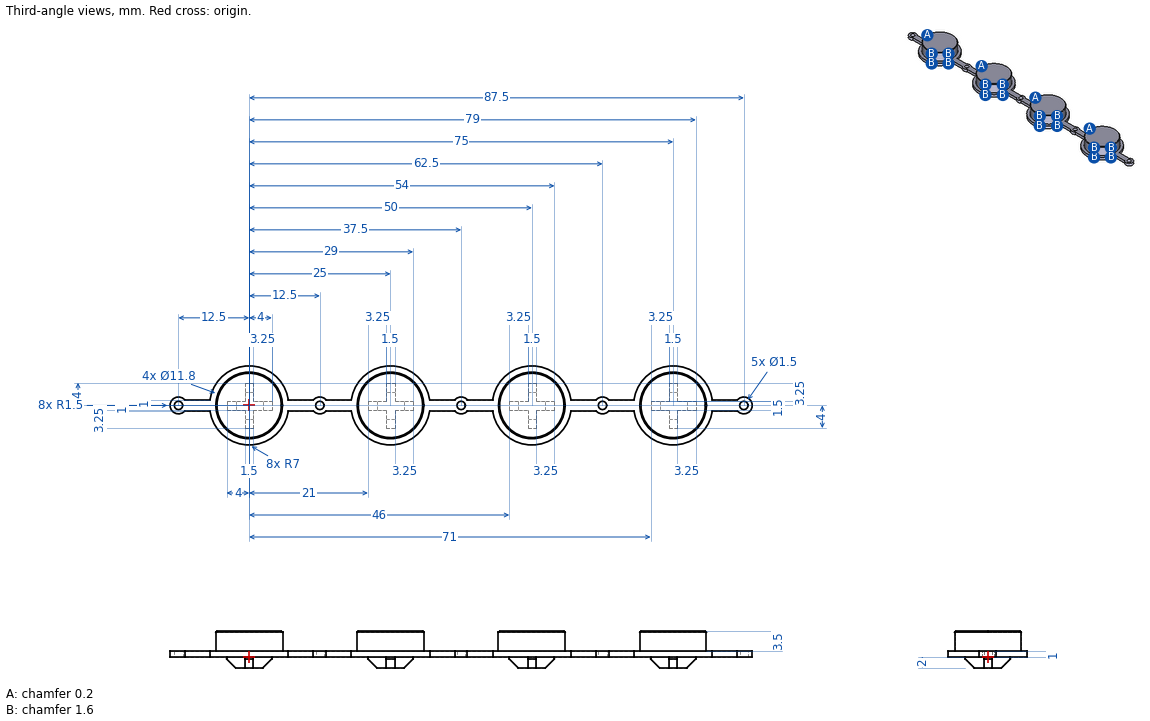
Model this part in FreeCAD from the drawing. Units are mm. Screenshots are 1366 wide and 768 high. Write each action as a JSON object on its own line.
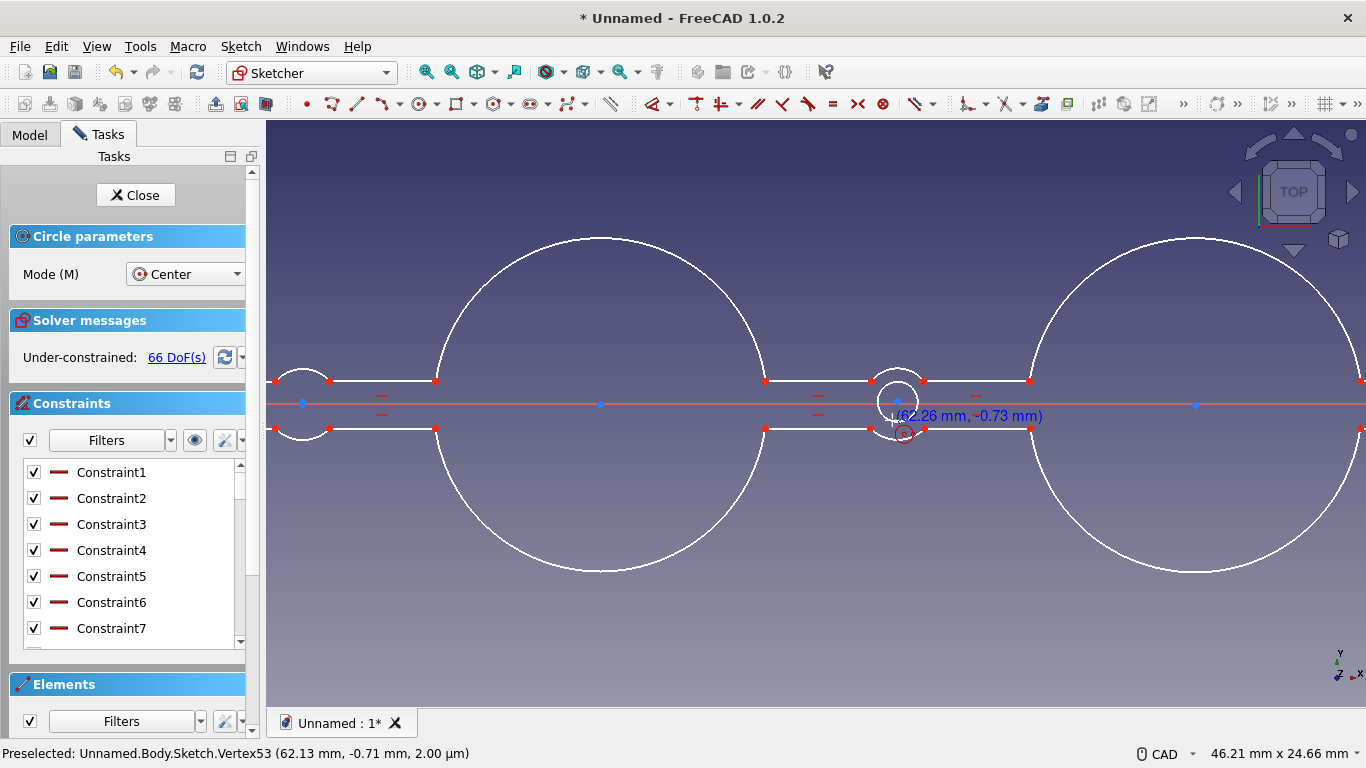
{"action": "scroll", "coordinate": [303, 404], "scroll_direction": "up", "scroll_amount": 2}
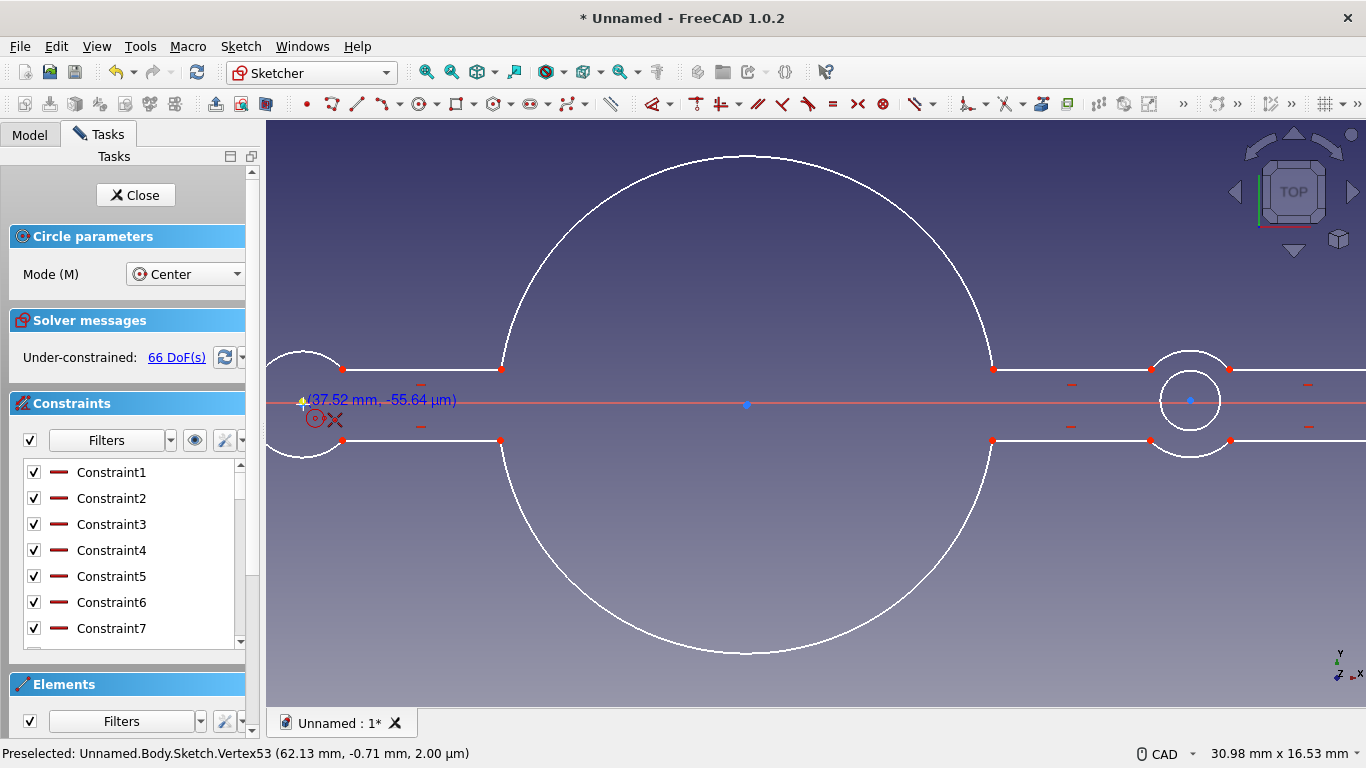
{"action": "scroll", "coordinate": [836, 416], "scroll_direction": "down", "scroll_amount": 9}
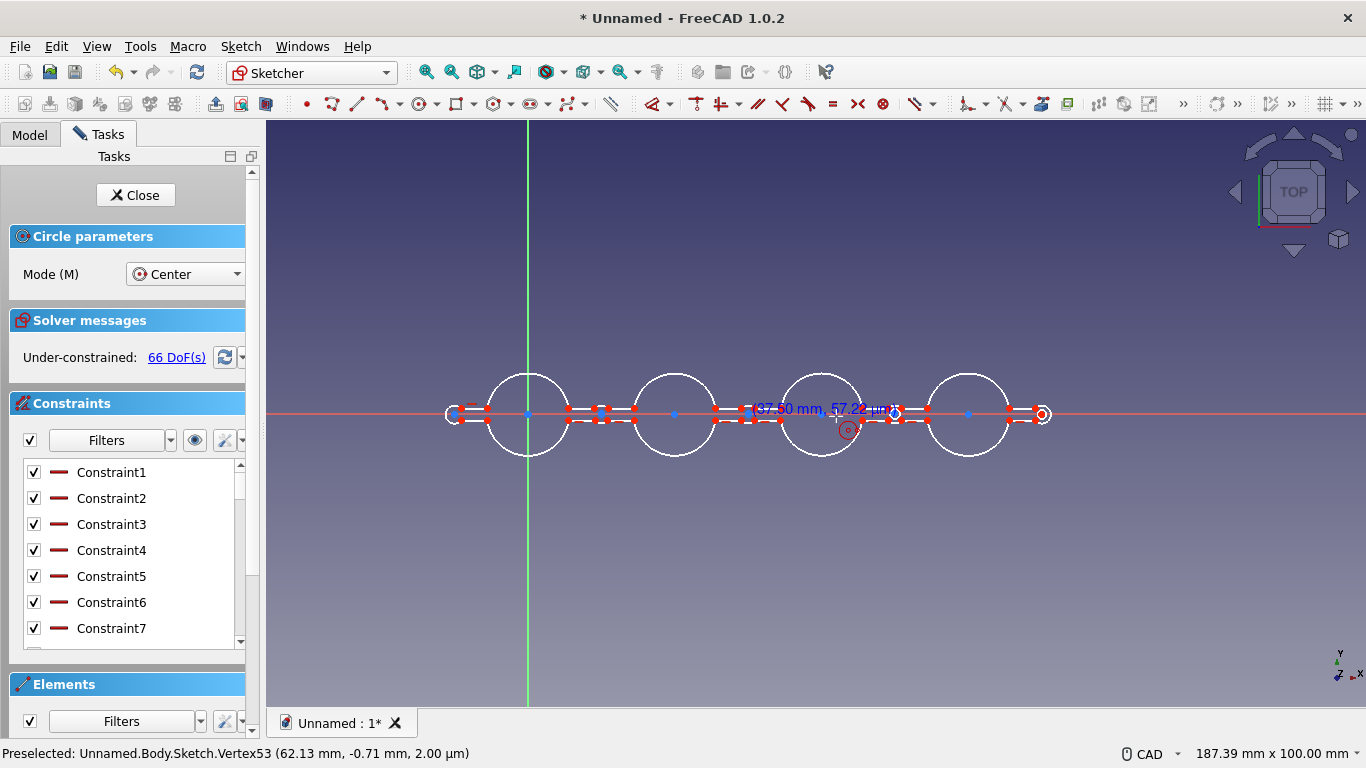
{"action": "scroll", "coordinate": [748, 414], "scroll_direction": "up", "scroll_amount": 3}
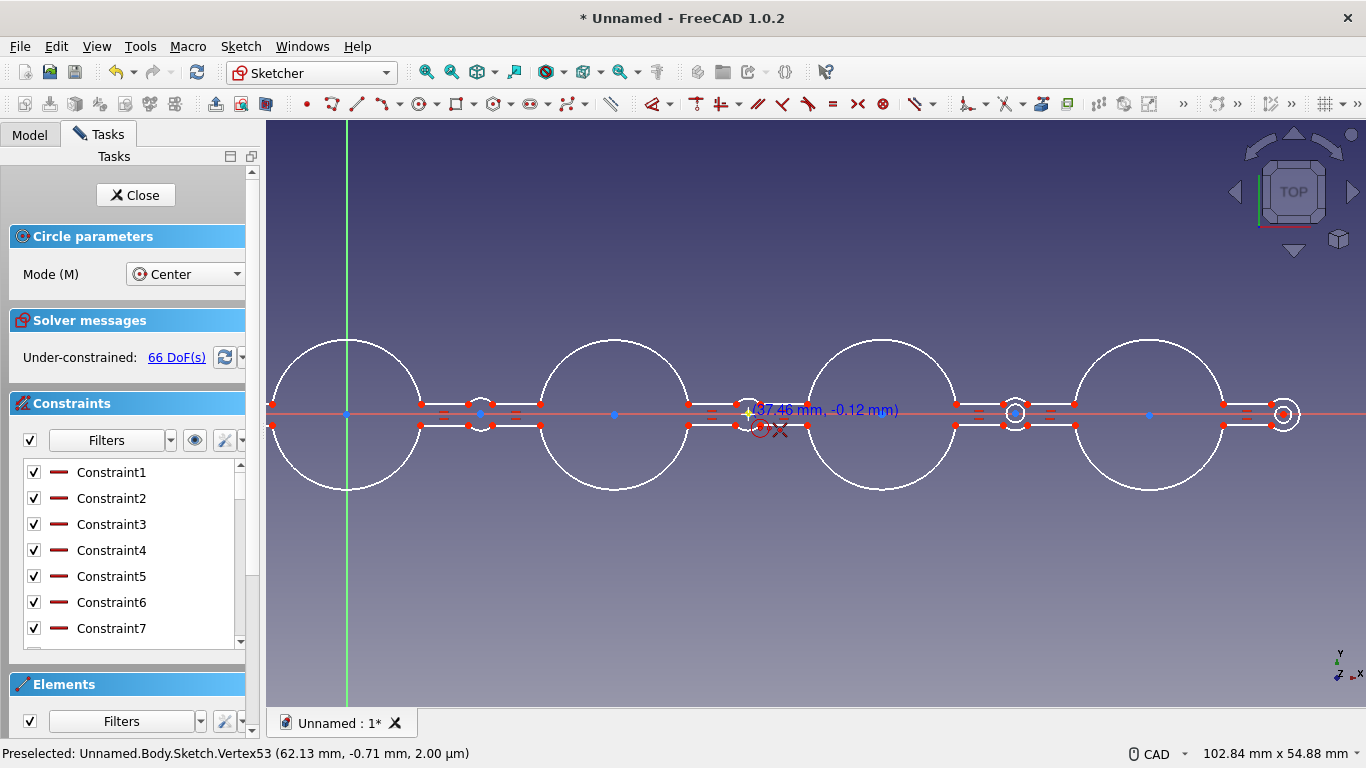
{"action": "left_click", "coordinate": [748, 414]}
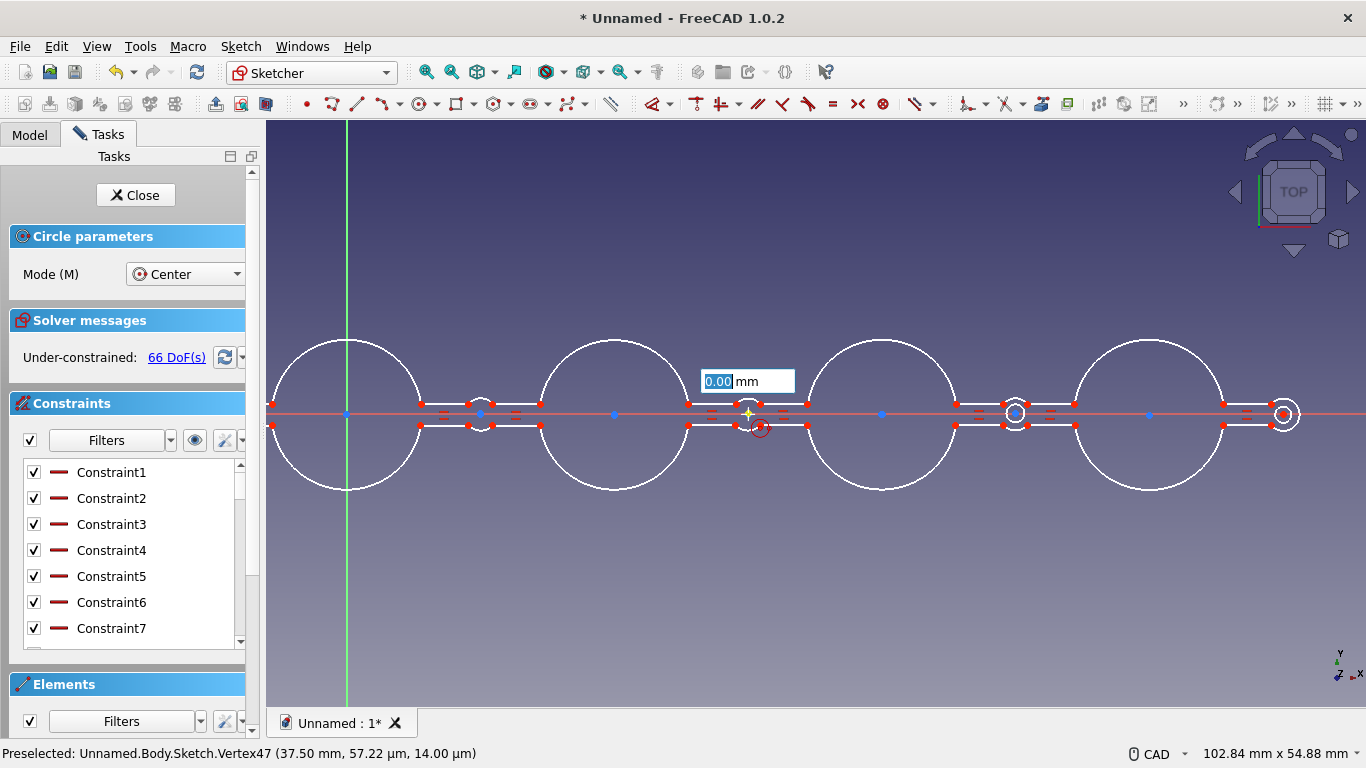
{"action": "scroll", "coordinate": [745, 422], "scroll_direction": "up", "scroll_amount": 4}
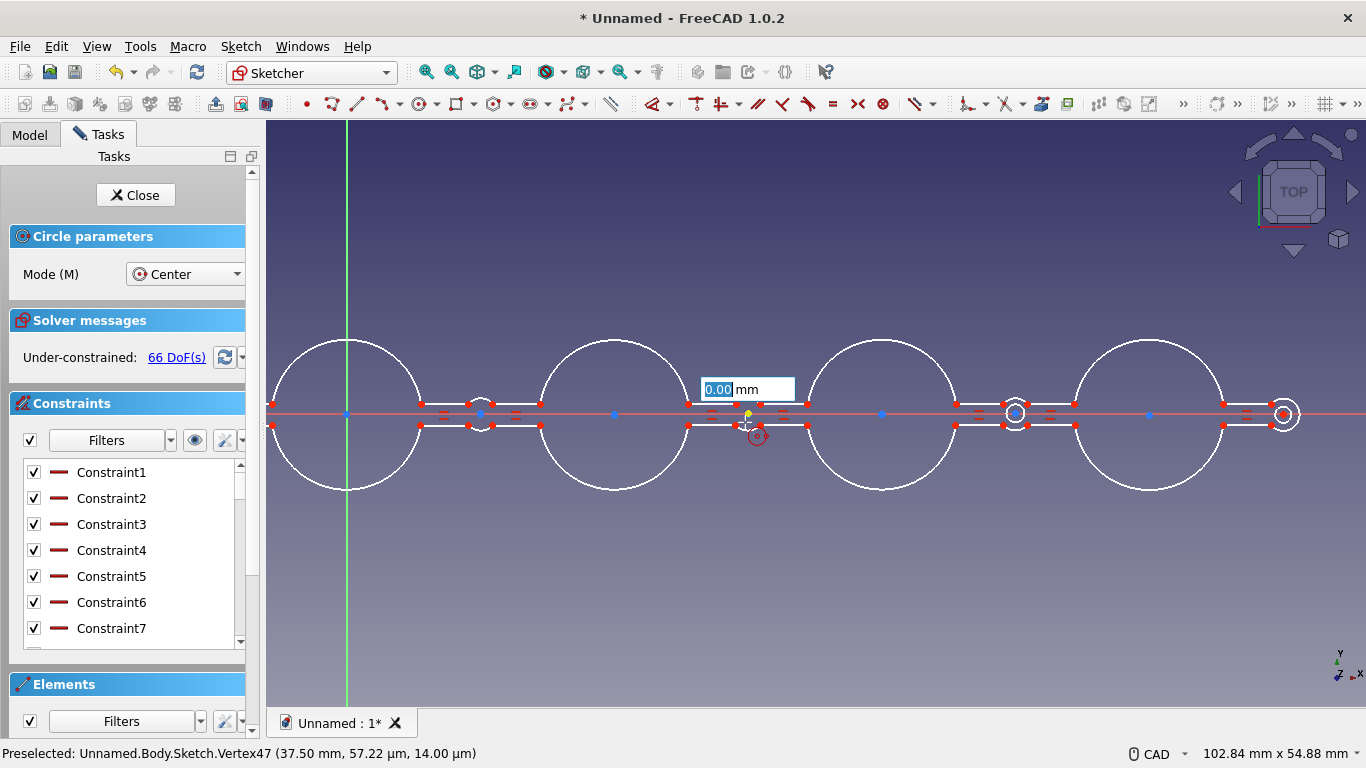
{"action": "left_click", "coordinate": [745, 421]}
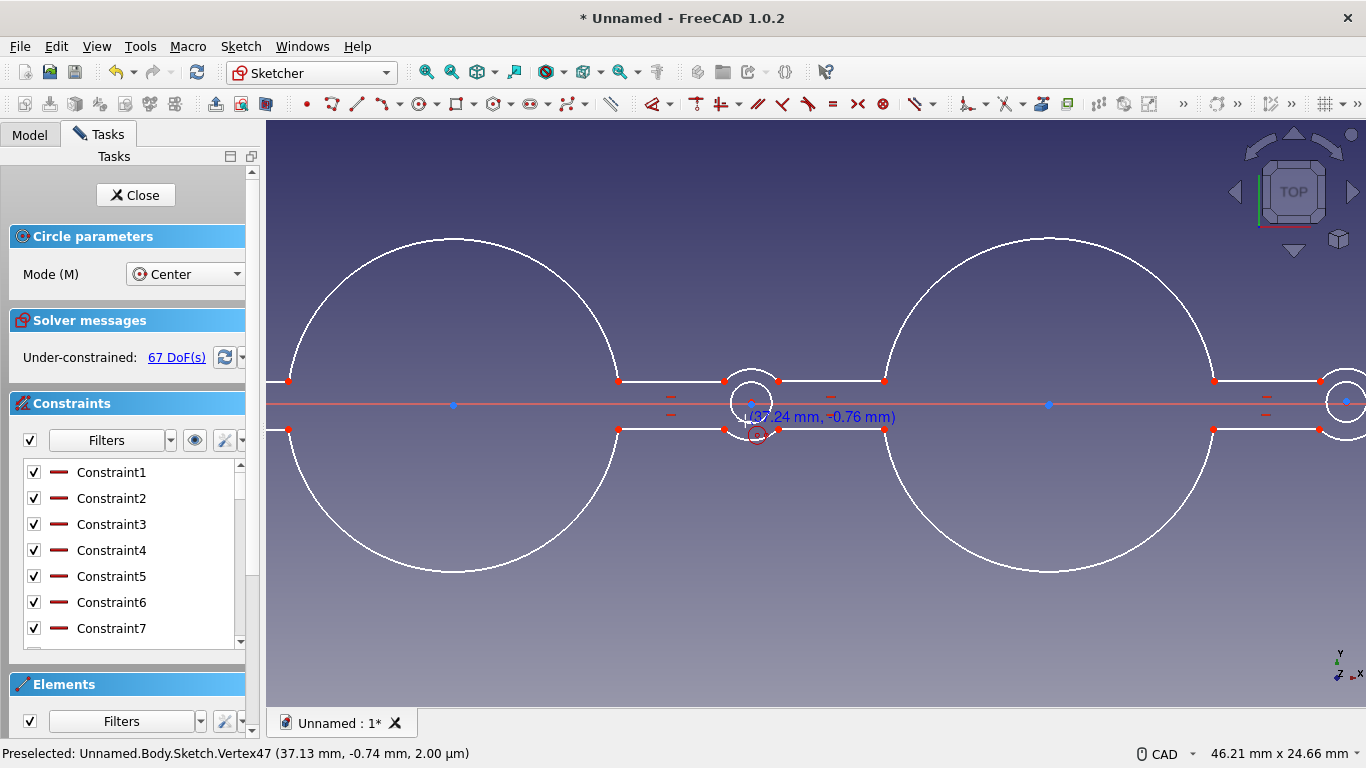
{"action": "scroll", "coordinate": [746, 417], "scroll_direction": "down", "scroll_amount": 7}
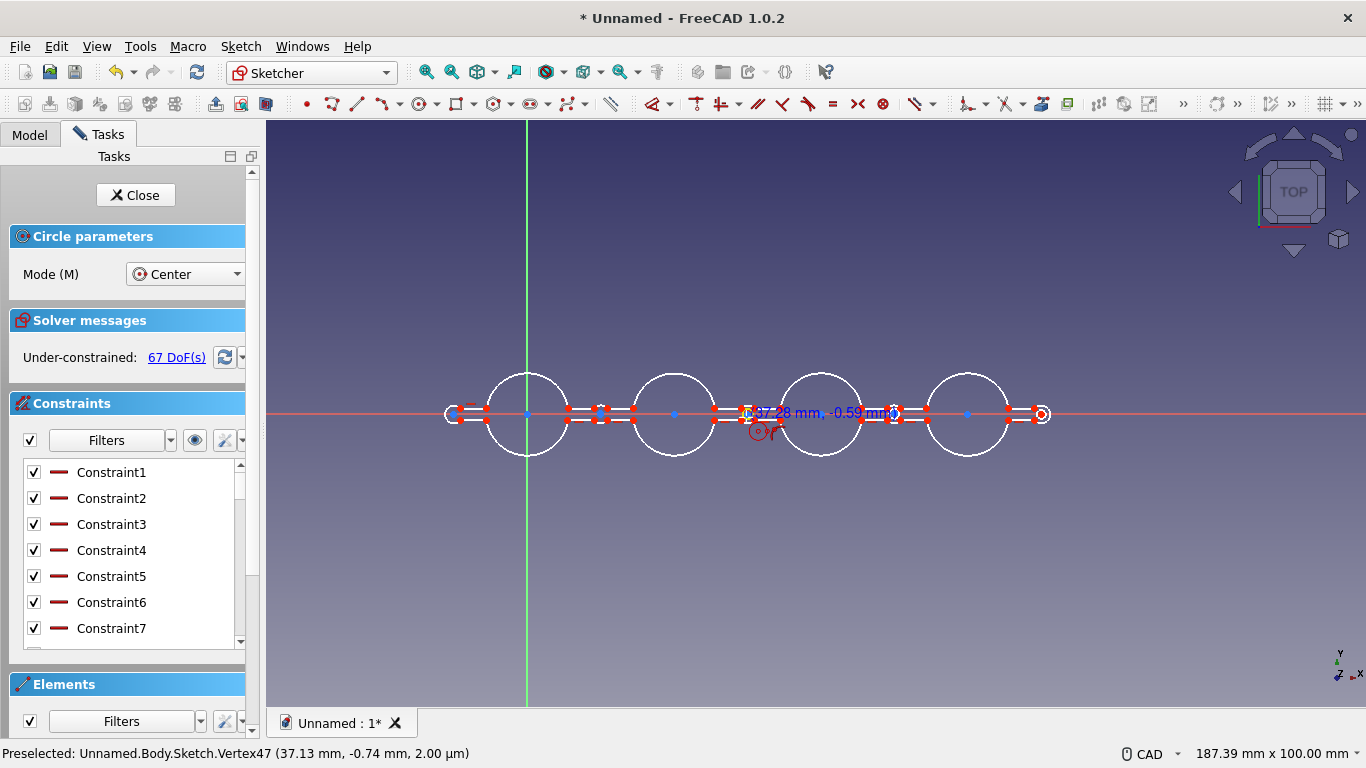
{"action": "scroll", "coordinate": [601, 414], "scroll_direction": "up", "scroll_amount": 9}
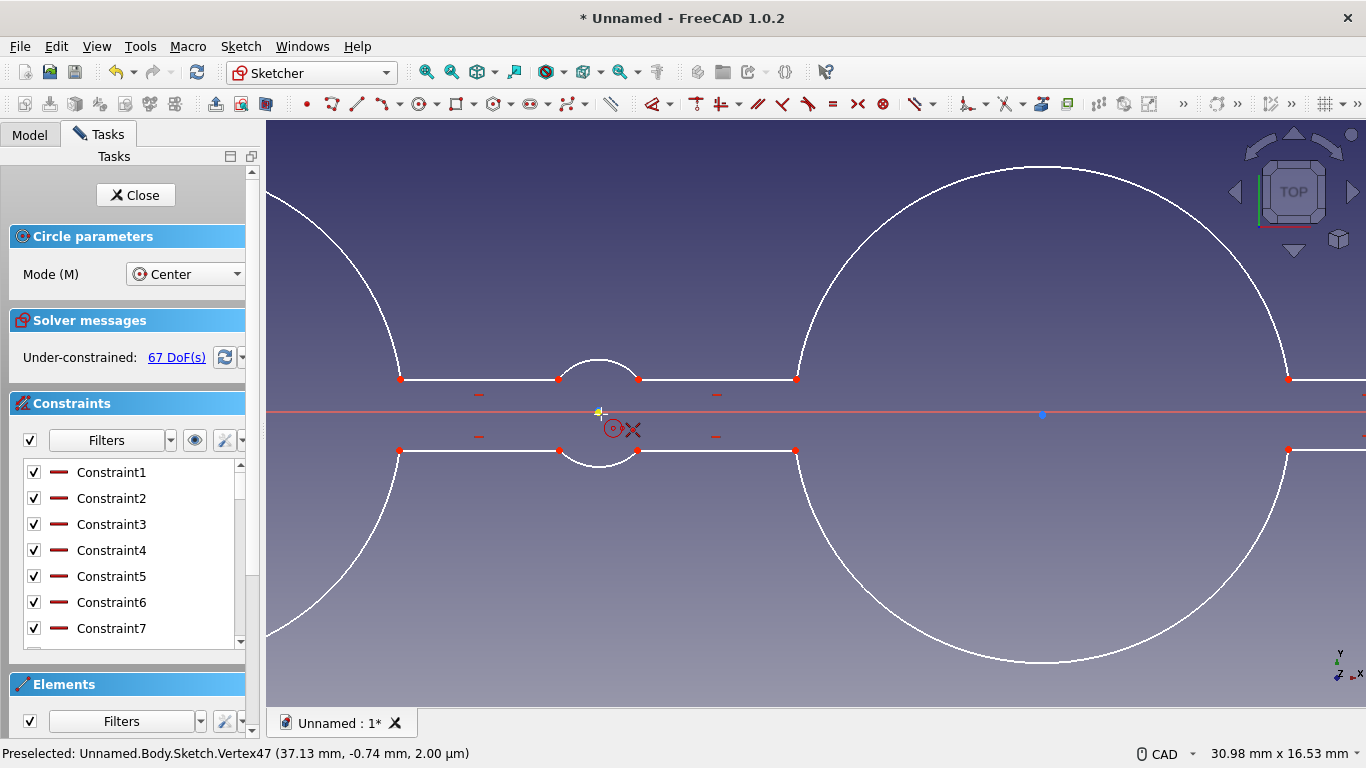
{"action": "scroll", "coordinate": [601, 414], "scroll_direction": "down", "scroll_amount": 9}